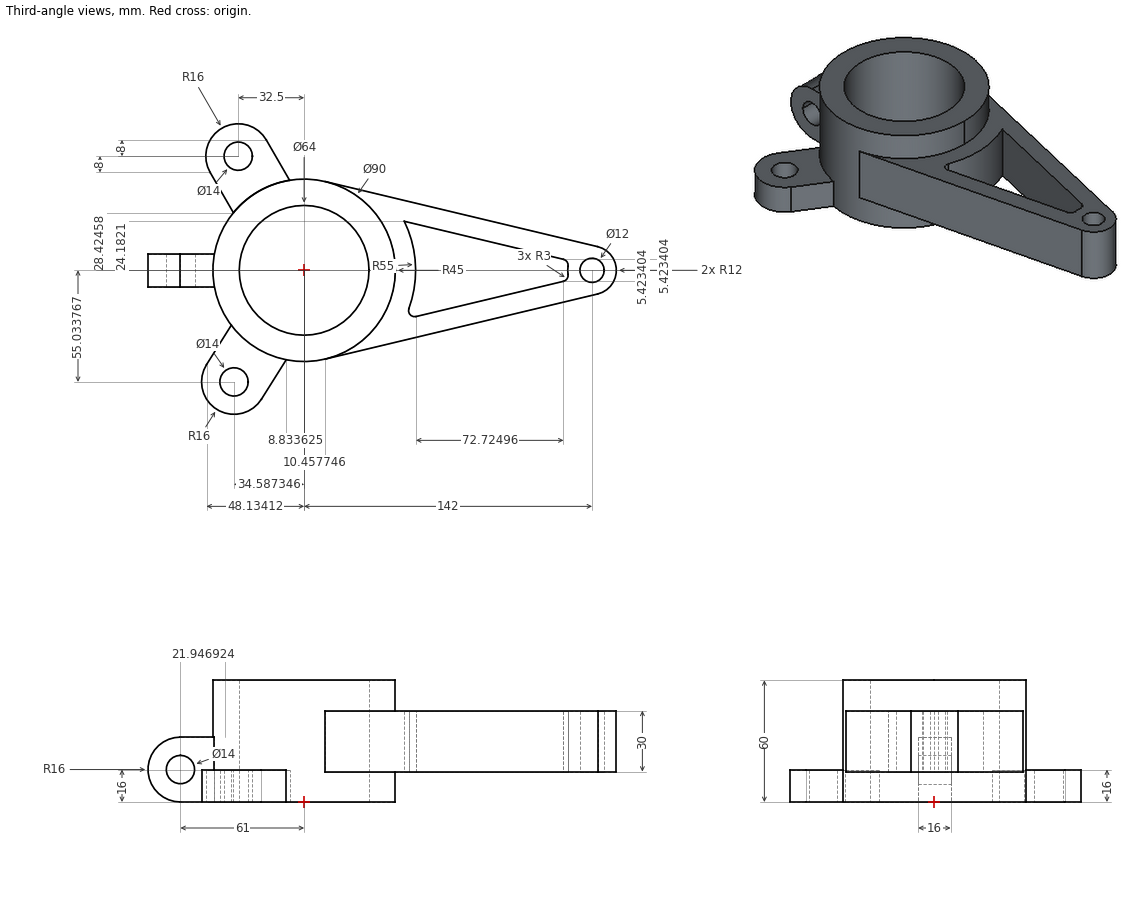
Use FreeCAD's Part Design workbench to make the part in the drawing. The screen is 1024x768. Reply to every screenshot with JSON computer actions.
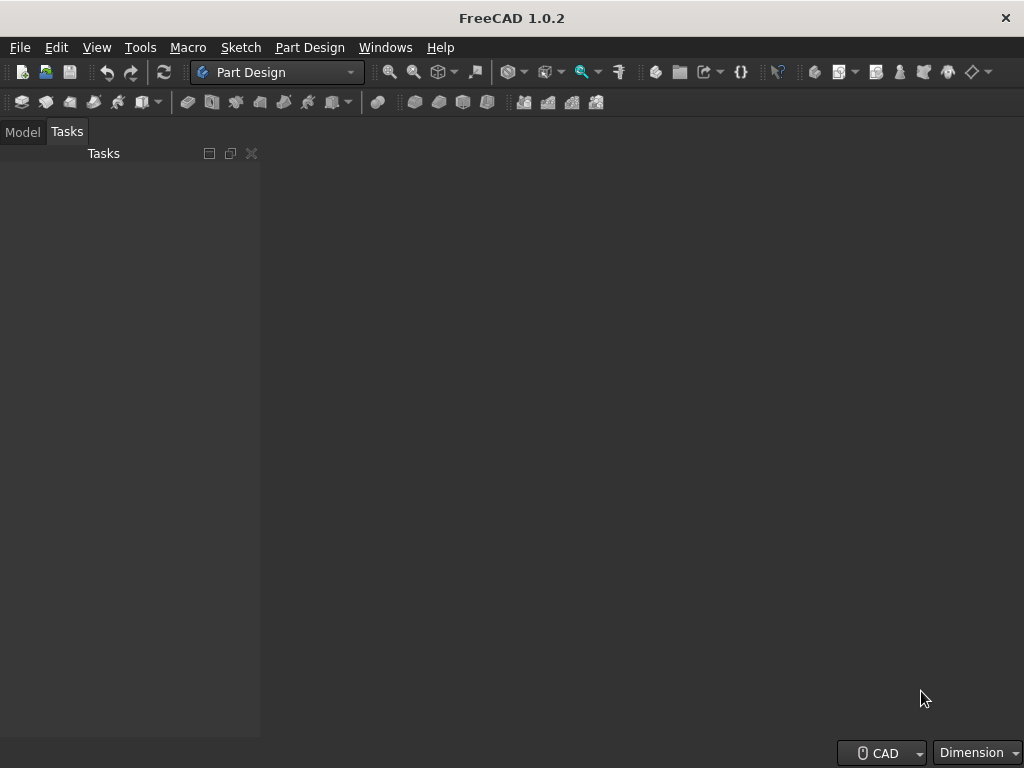
{"action": "left_click", "coordinate": [22, 72]}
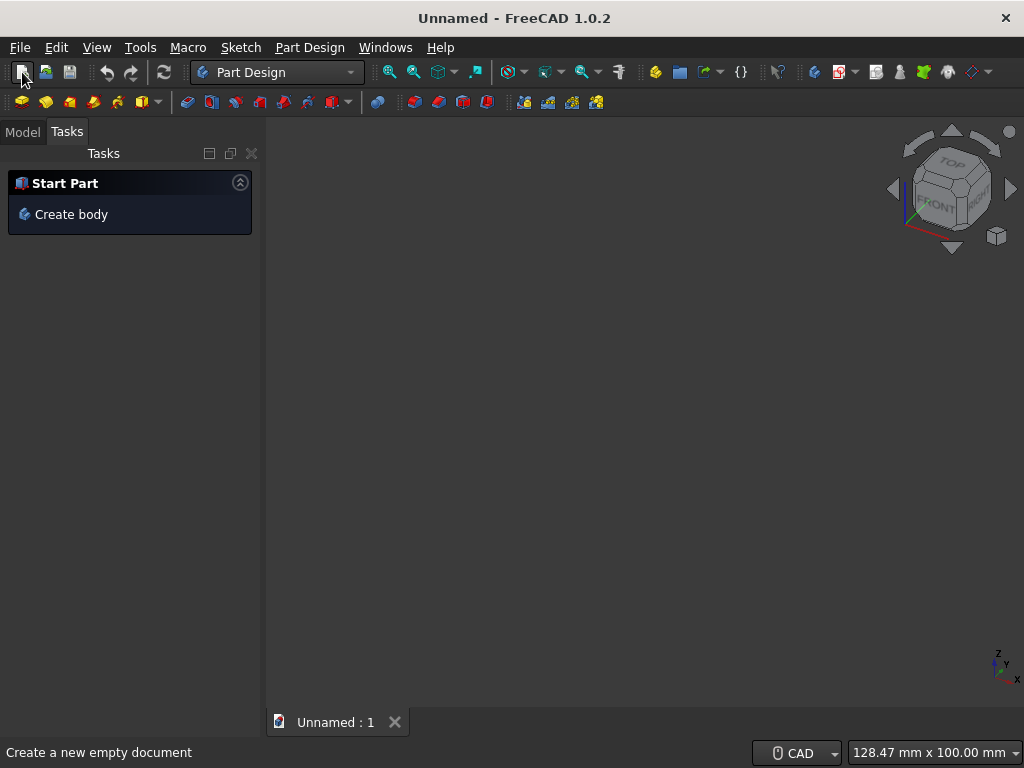
{"action": "left_click", "coordinate": [840, 72]}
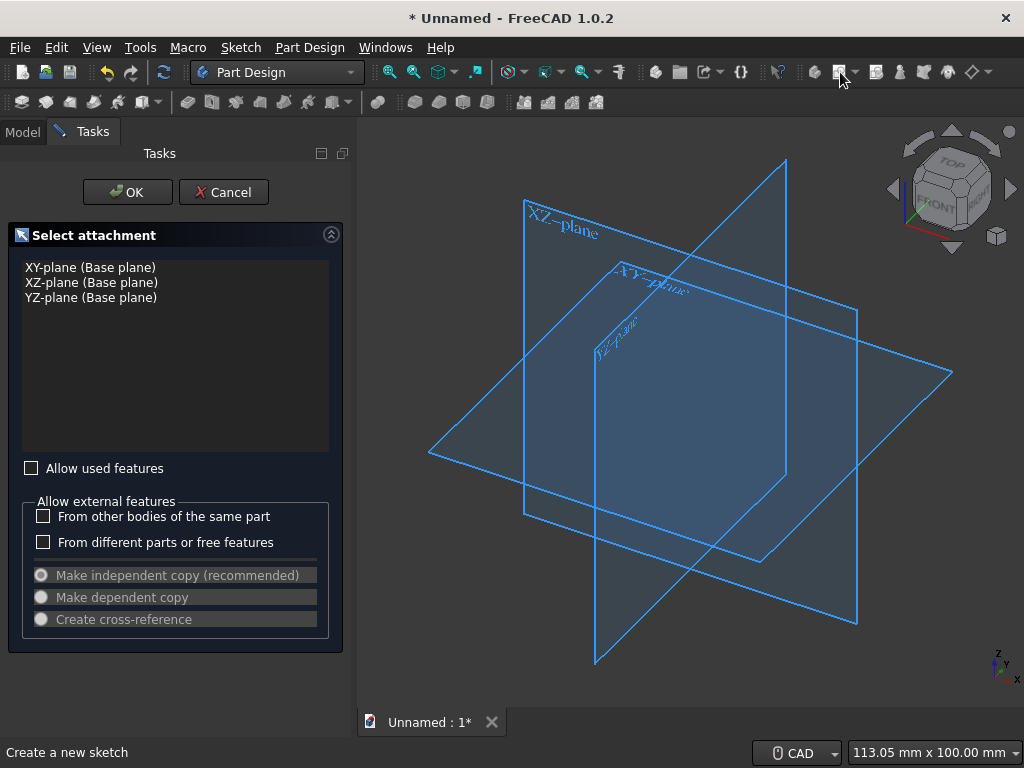
{"action": "left_click", "coordinate": [82, 268]}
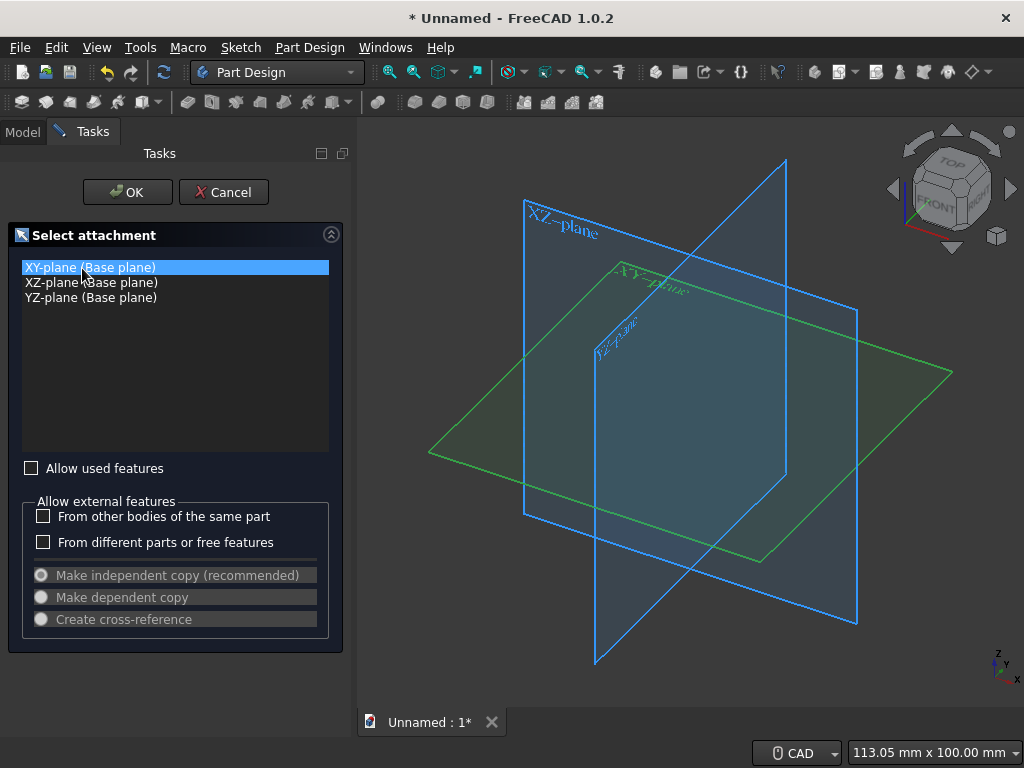
{"action": "left_click", "coordinate": [128, 192]}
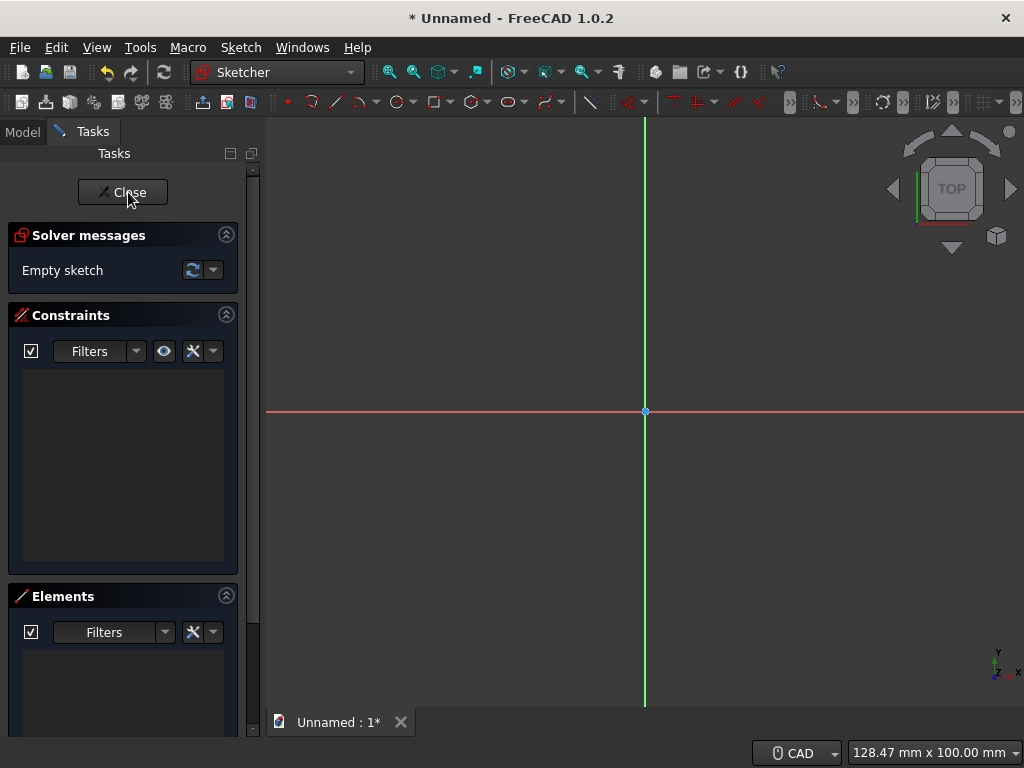
{"action": "scroll", "coordinate": [437, 412], "scroll_direction": "down", "scroll_amount": 2}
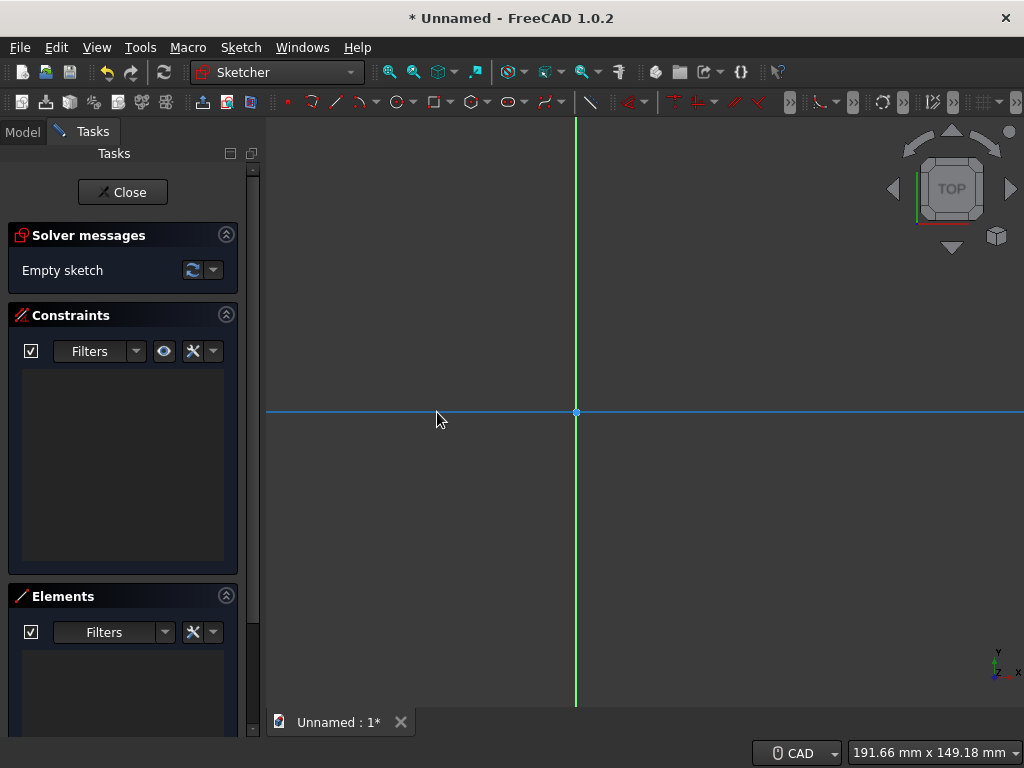
{"action": "key", "text": "g c"}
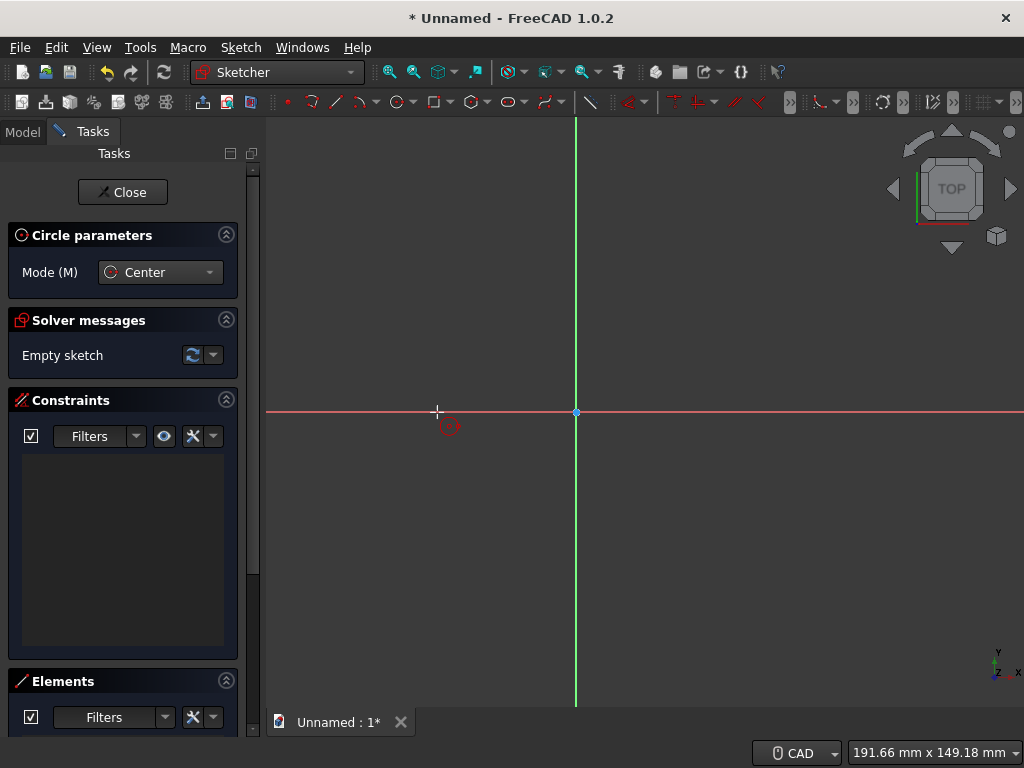
{"action": "left_click", "coordinate": [577, 412]}
{"action": "left_click", "coordinate": [702, 286]}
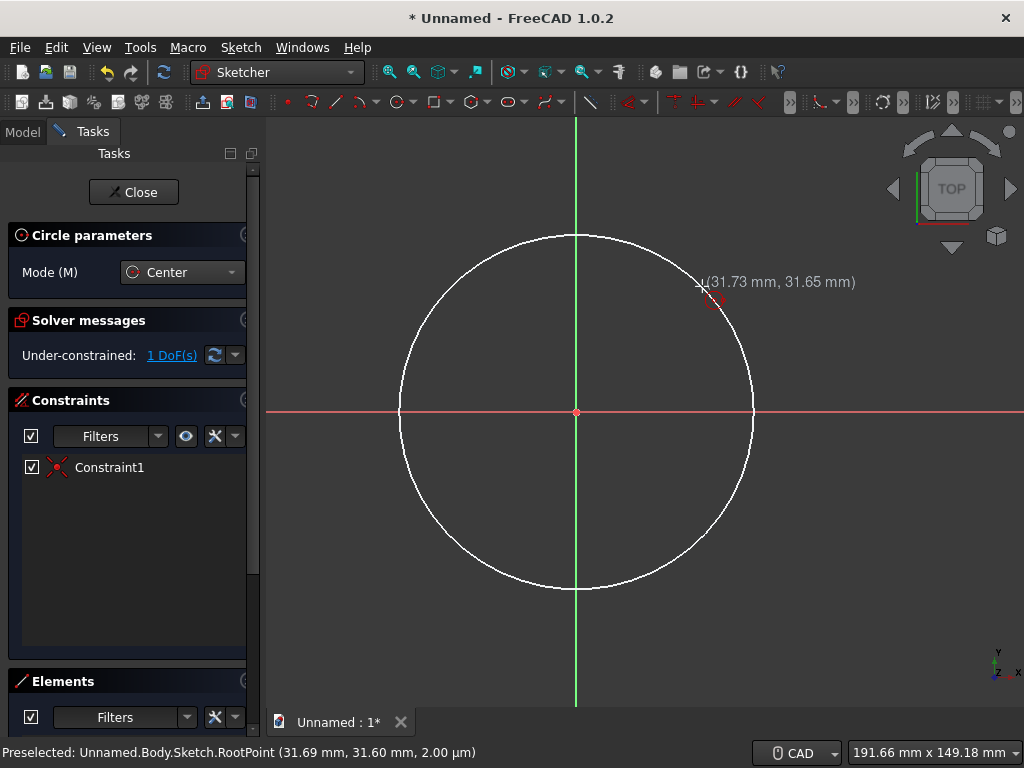
{"action": "left_click", "coordinate": [577, 412]}
{"action": "left_click", "coordinate": [666, 323]}
{"action": "key", "text": "Escape"}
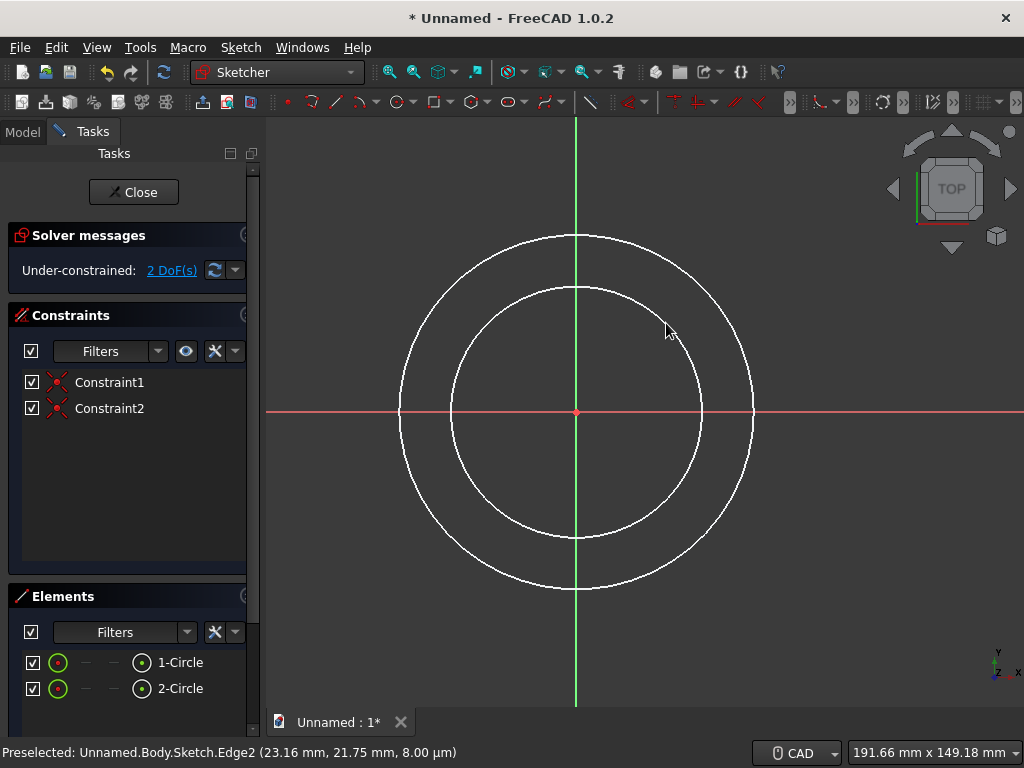
{"action": "key", "text": "d"}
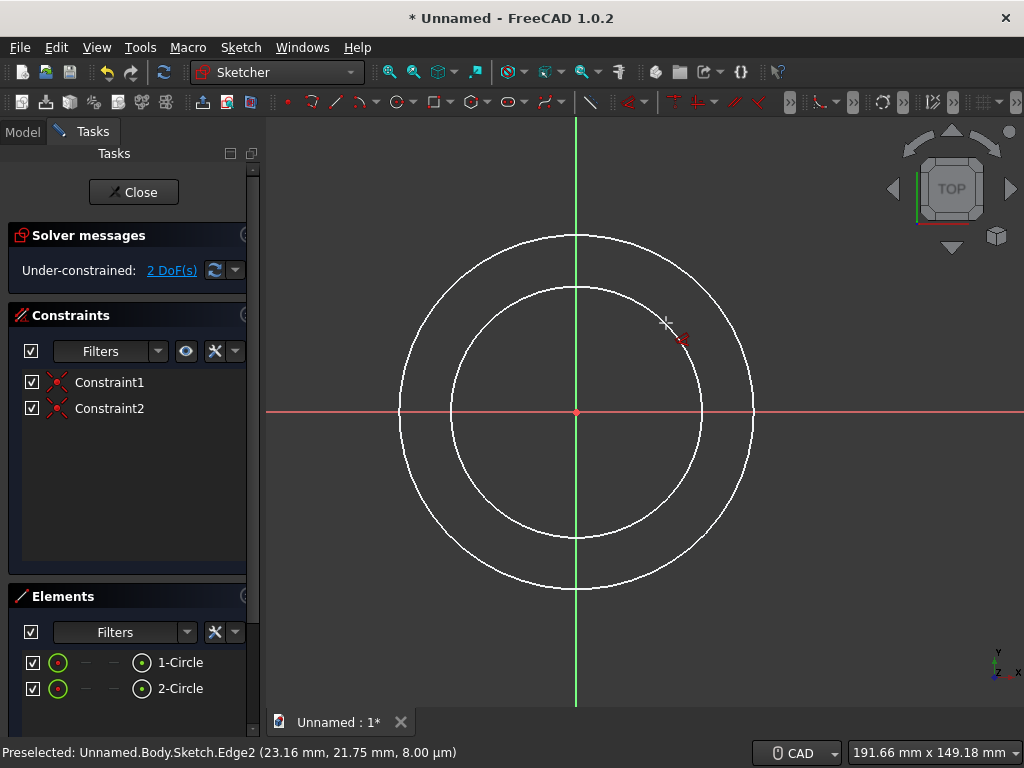
{"action": "left_click", "coordinate": [701, 286]}
{"action": "left_click", "coordinate": [723, 263]}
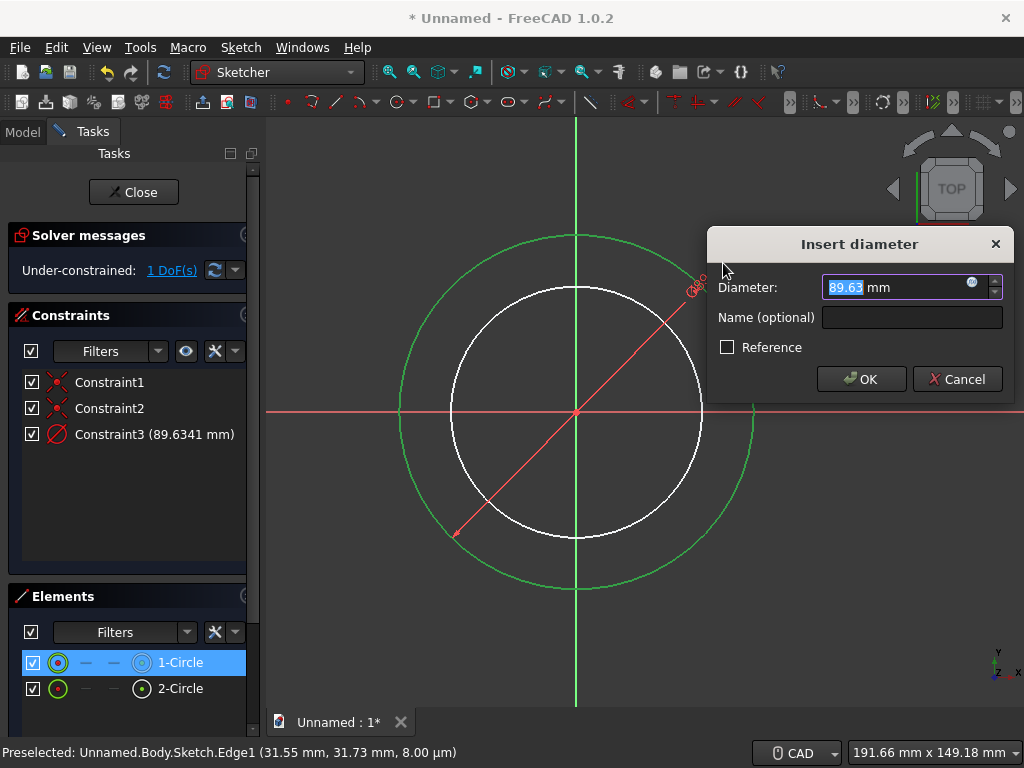
{"action": "type", "text": "90"}
{"action": "key", "text": "Return"}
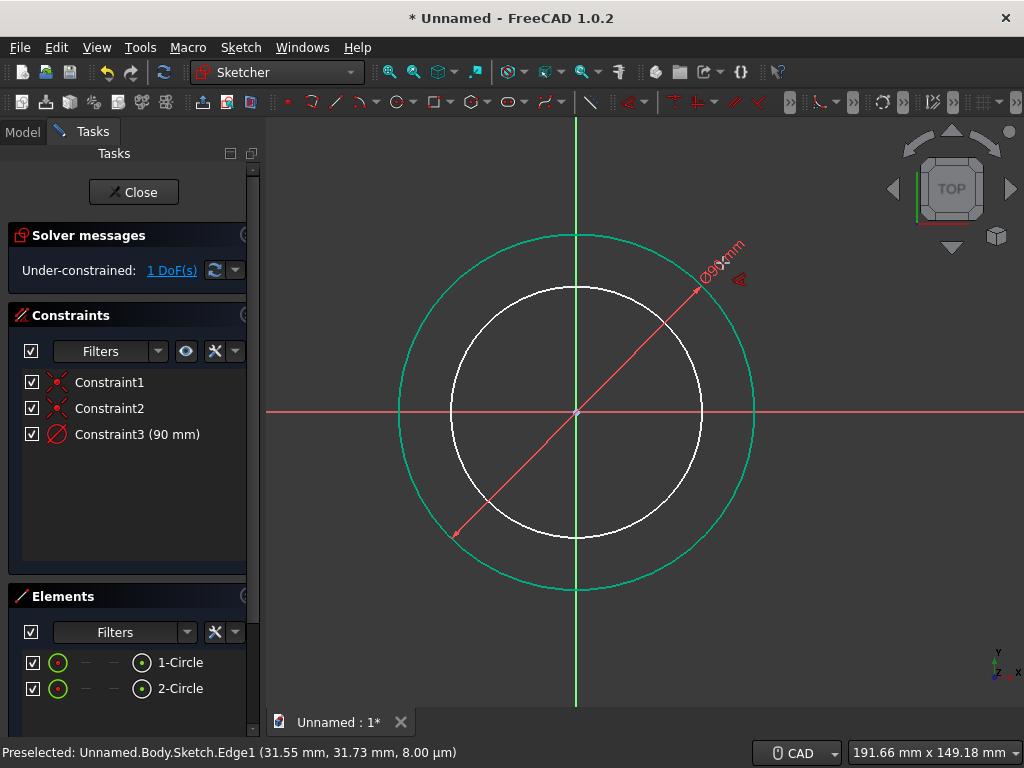
{"action": "left_click", "coordinate": [665, 323]}
{"action": "left_click", "coordinate": [688, 300]}